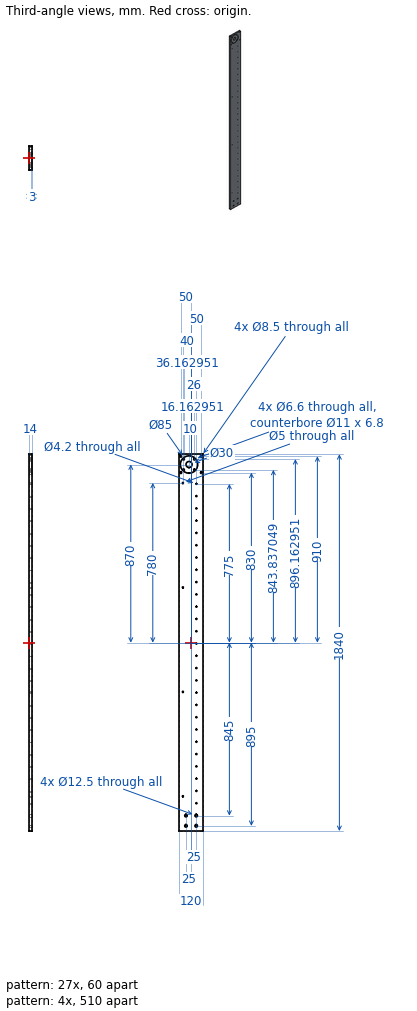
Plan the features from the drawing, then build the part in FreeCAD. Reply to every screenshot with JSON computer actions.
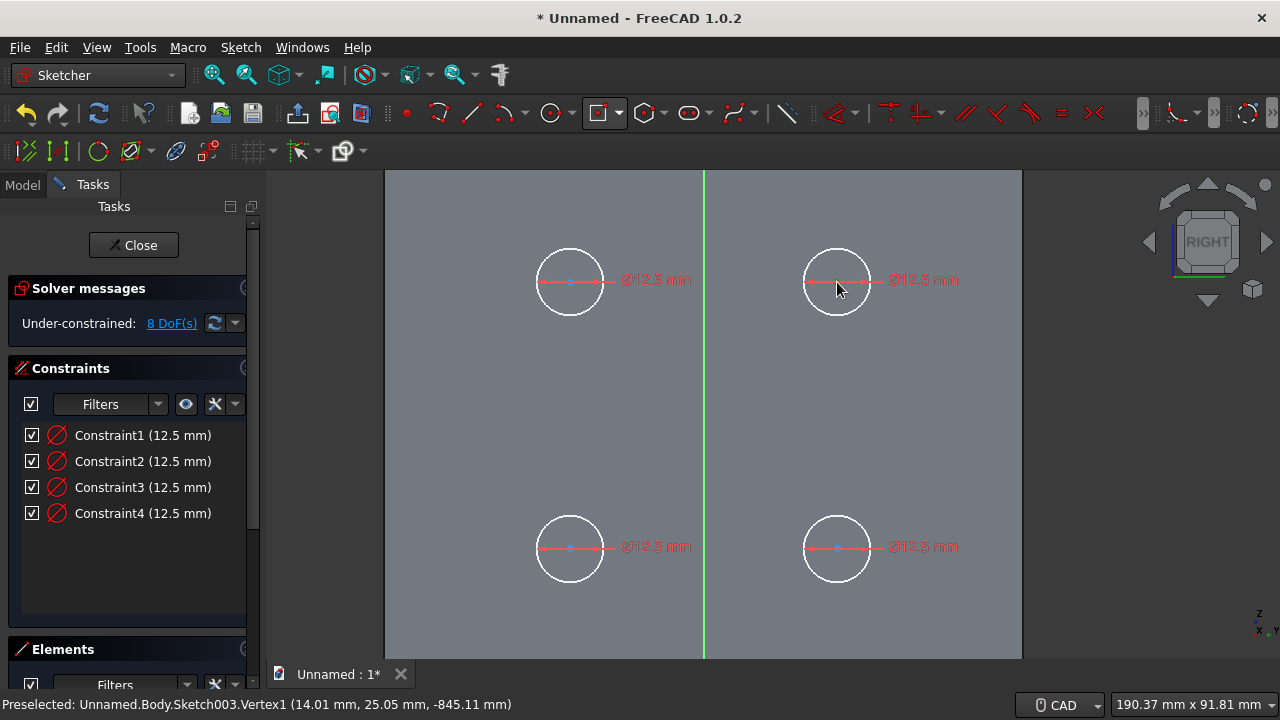
{"action": "left_click", "coordinate": [837, 549]}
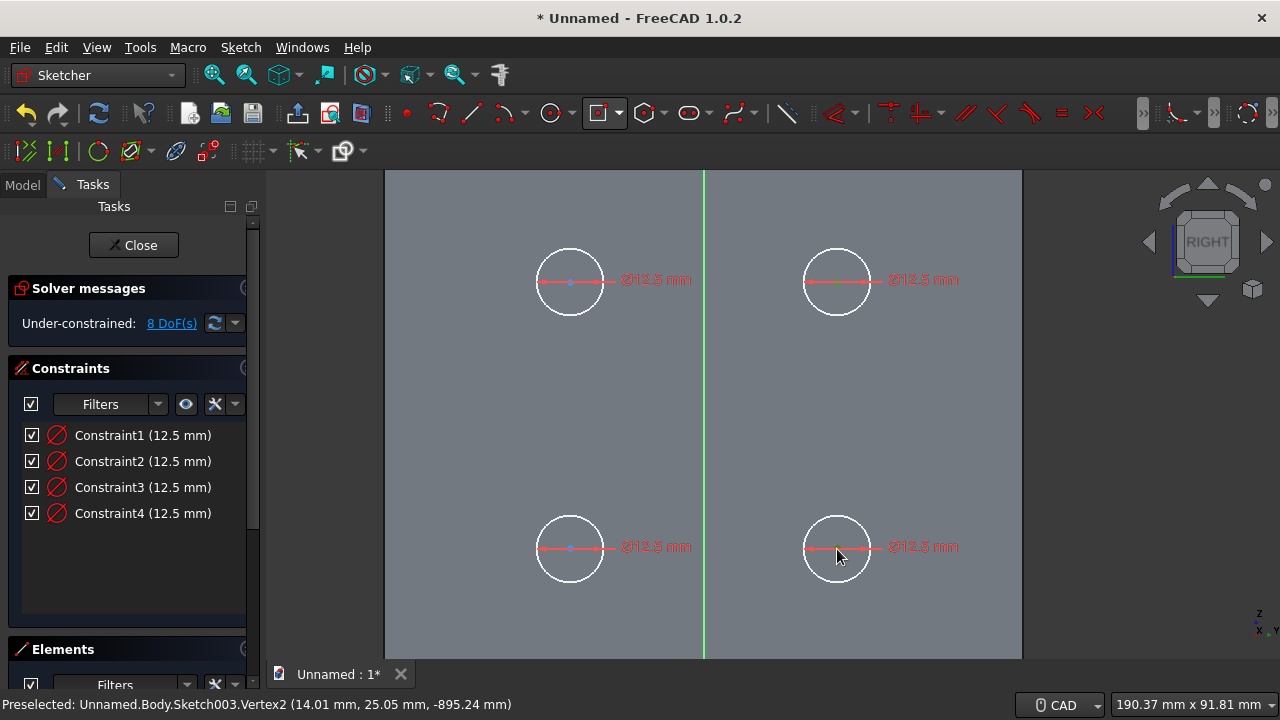
{"action": "left_click", "coordinate": [944, 114]}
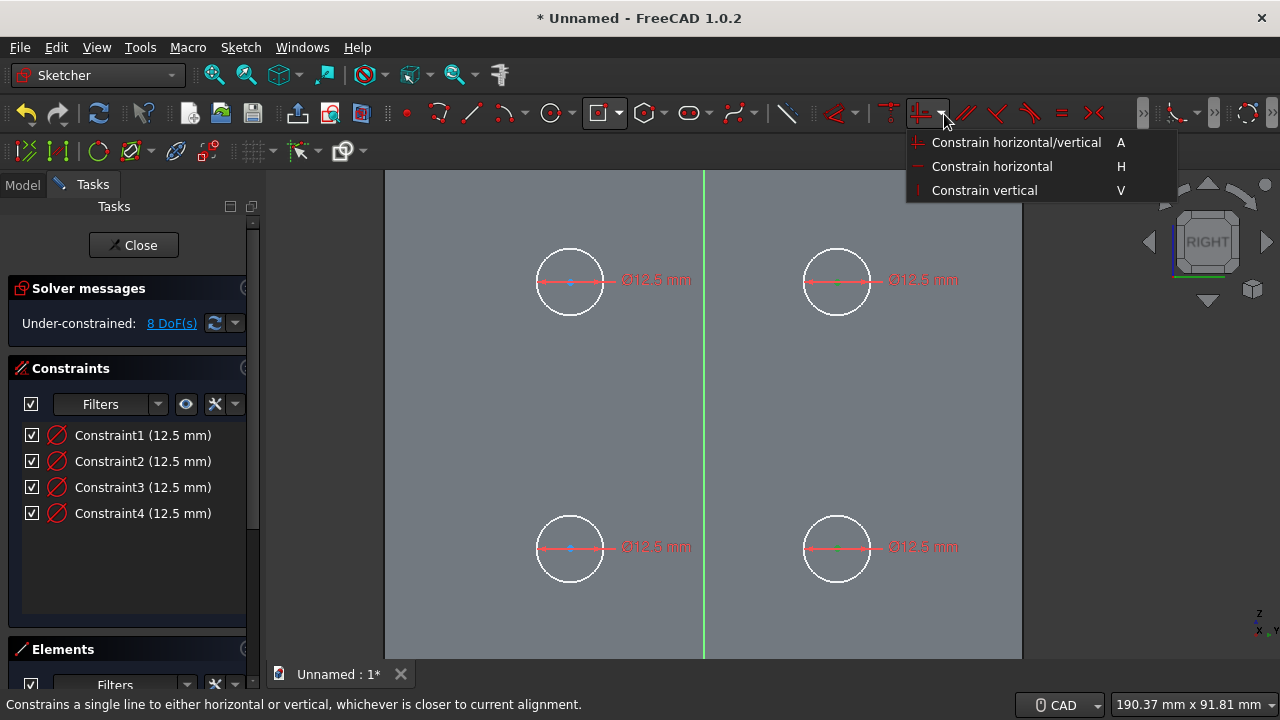
{"action": "left_click", "coordinate": [1042, 190]}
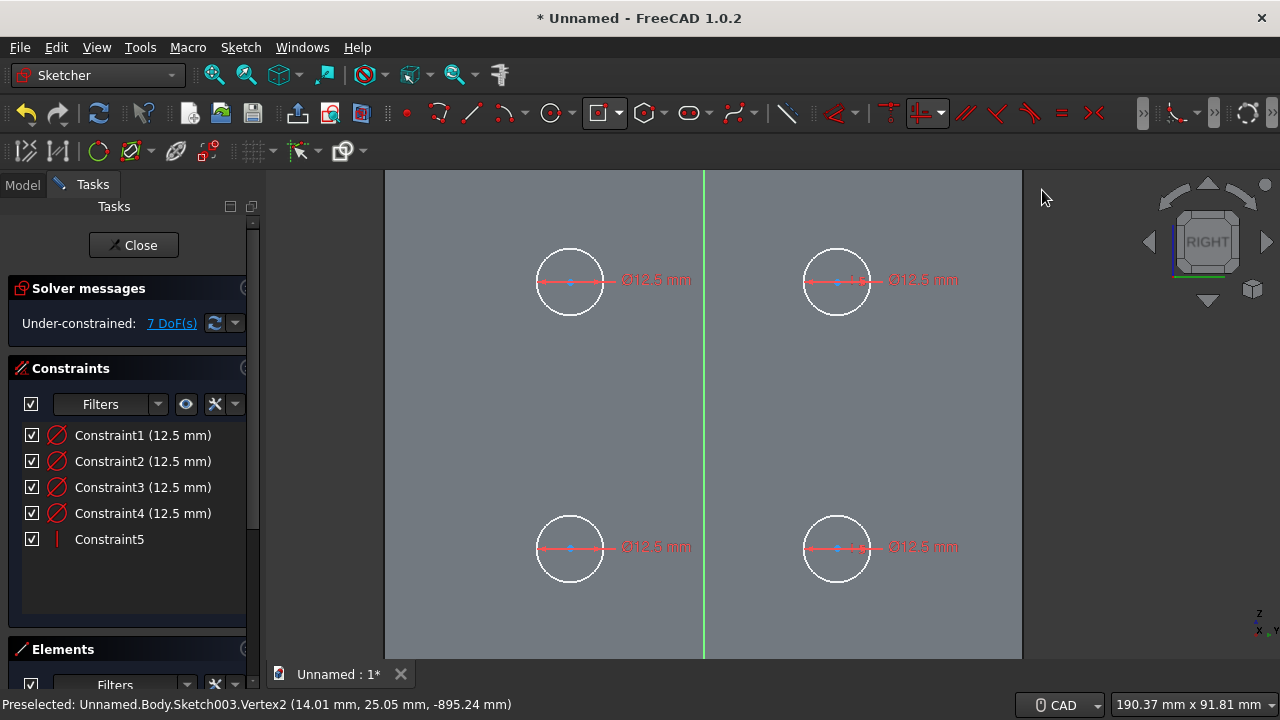
{"action": "left_click", "coordinate": [837, 282]}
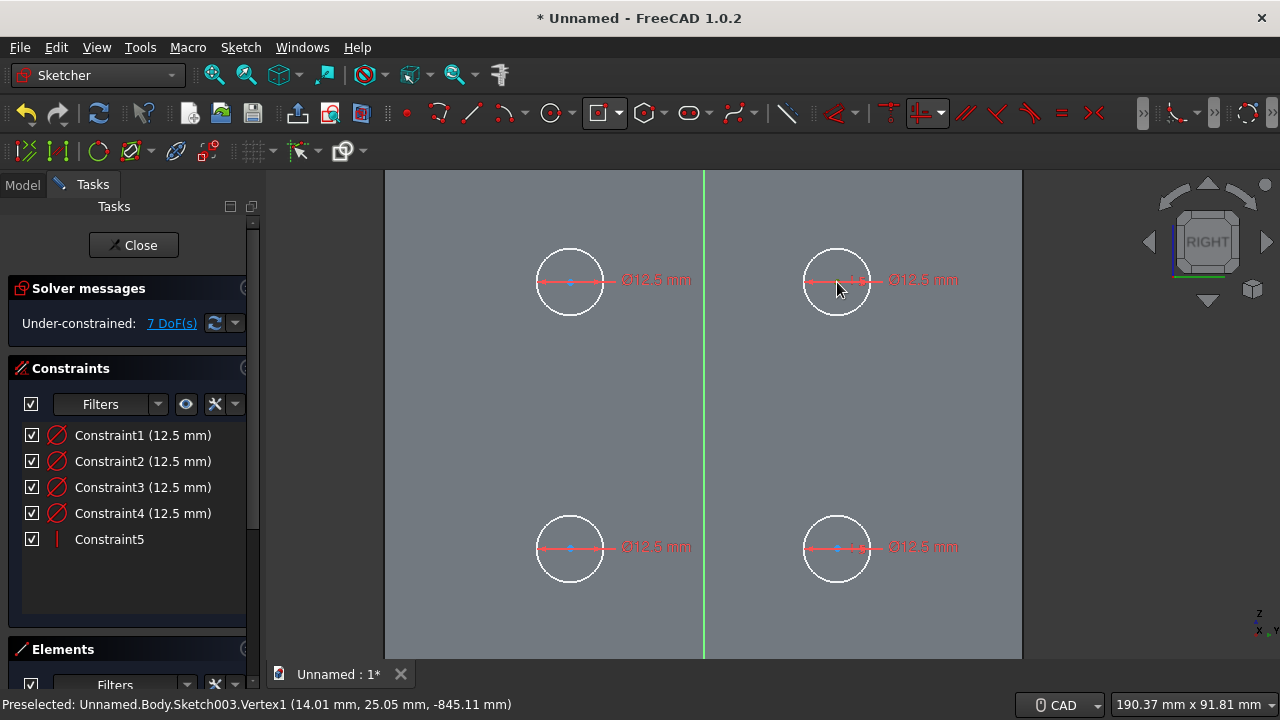
{"action": "left_click", "coordinate": [570, 282]}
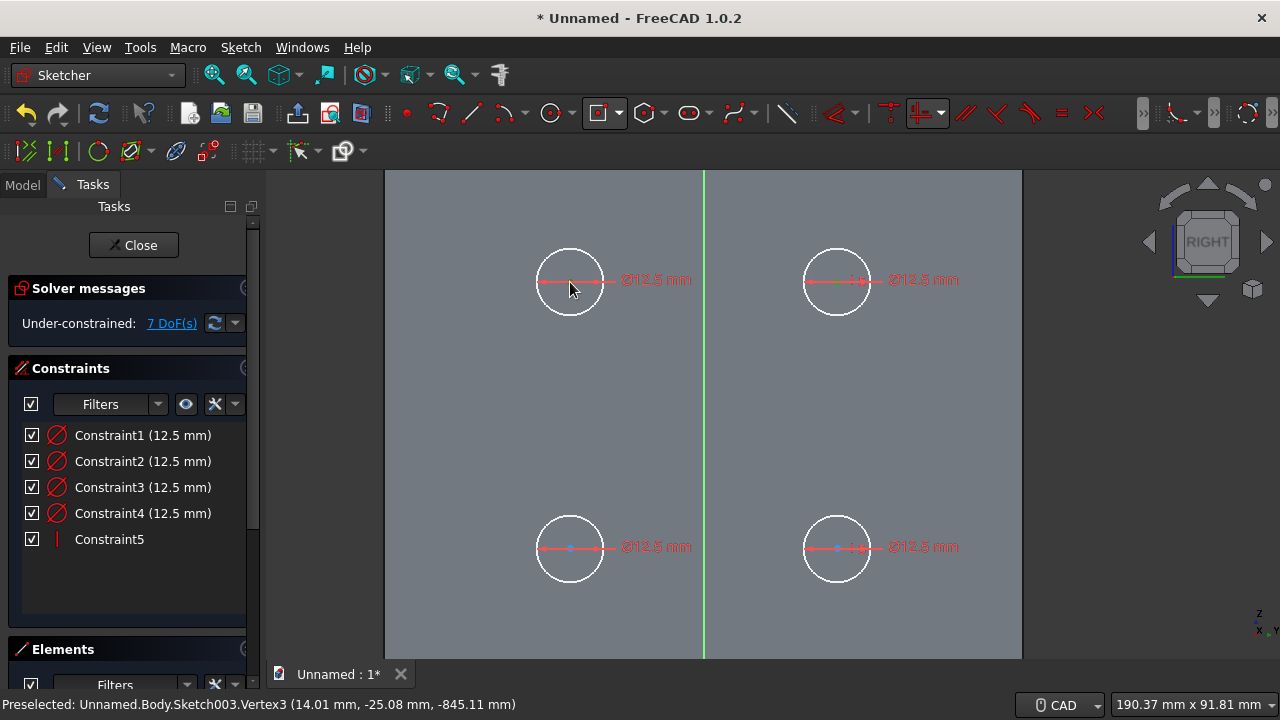
{"action": "key", "text": "h"}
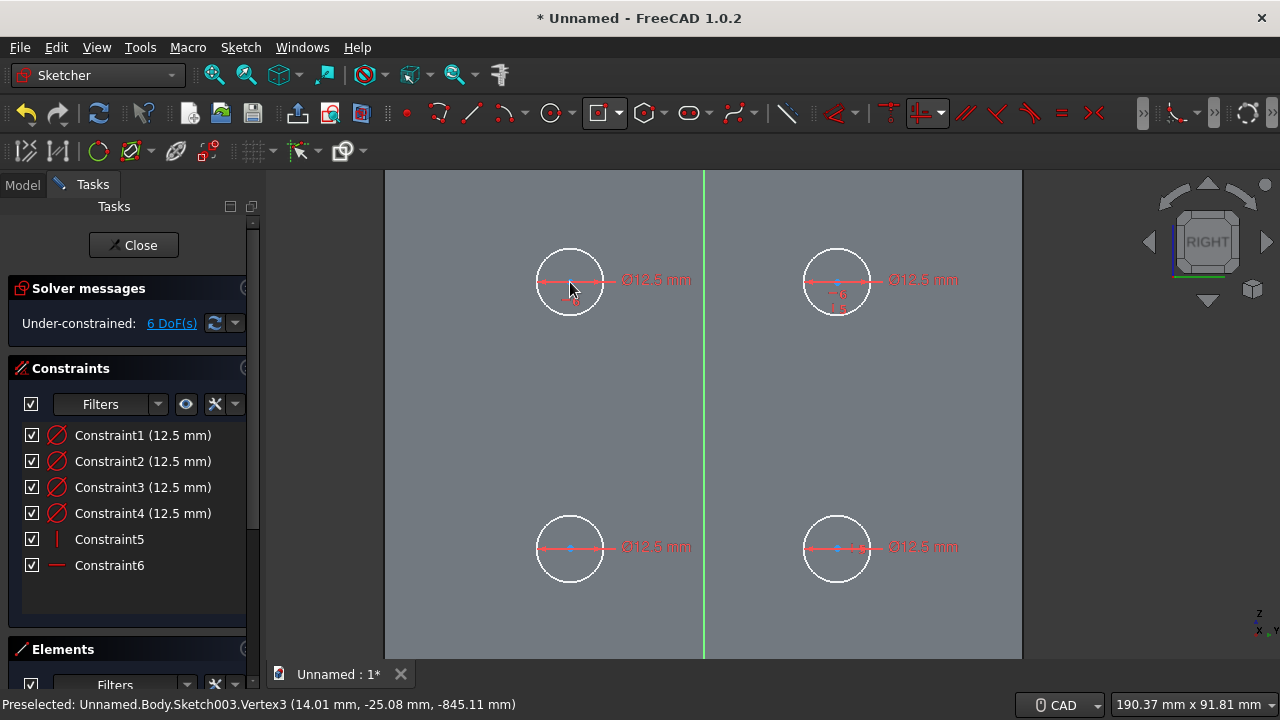
{"action": "left_click", "coordinate": [570, 282]}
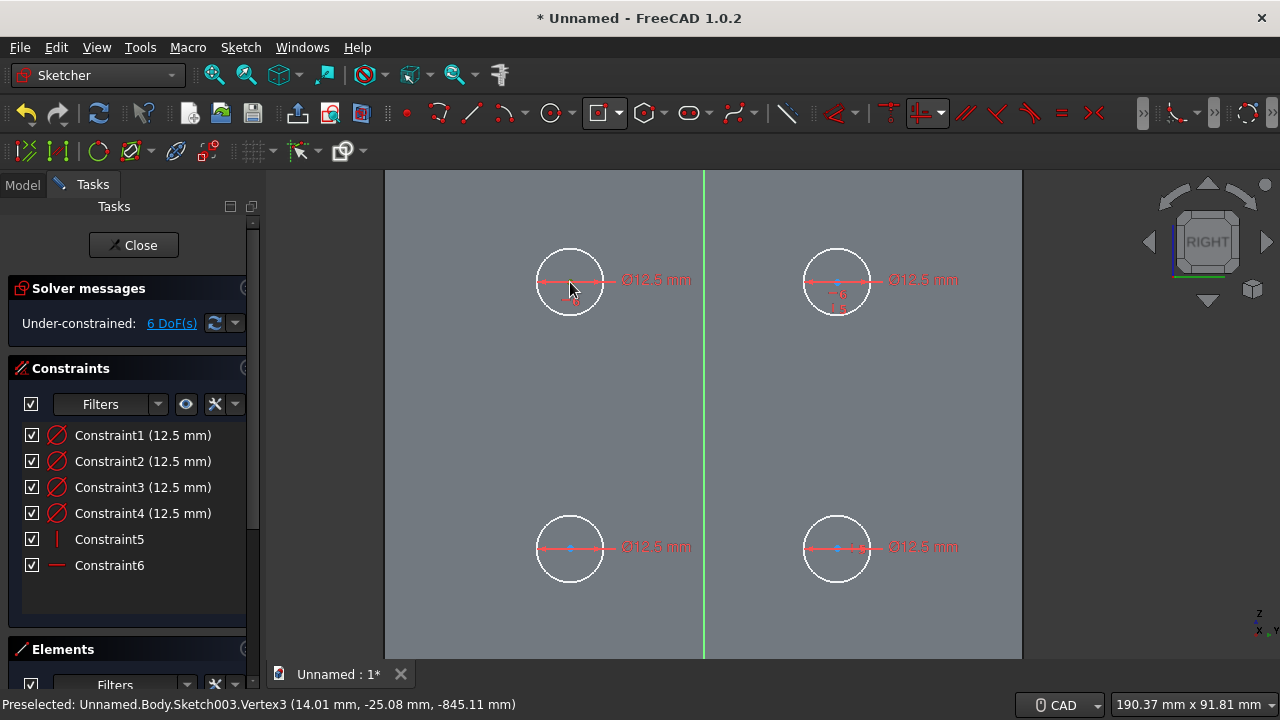
{"action": "left_click", "coordinate": [570, 549]}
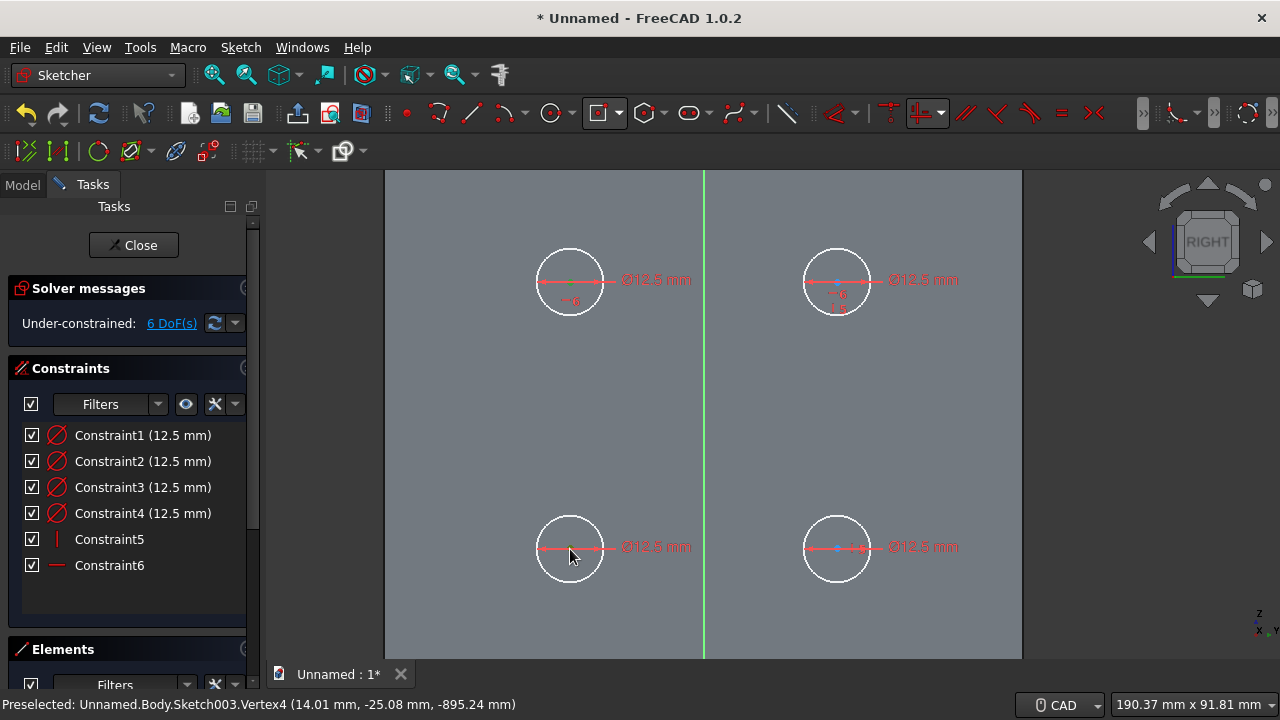
{"action": "key", "text": "v"}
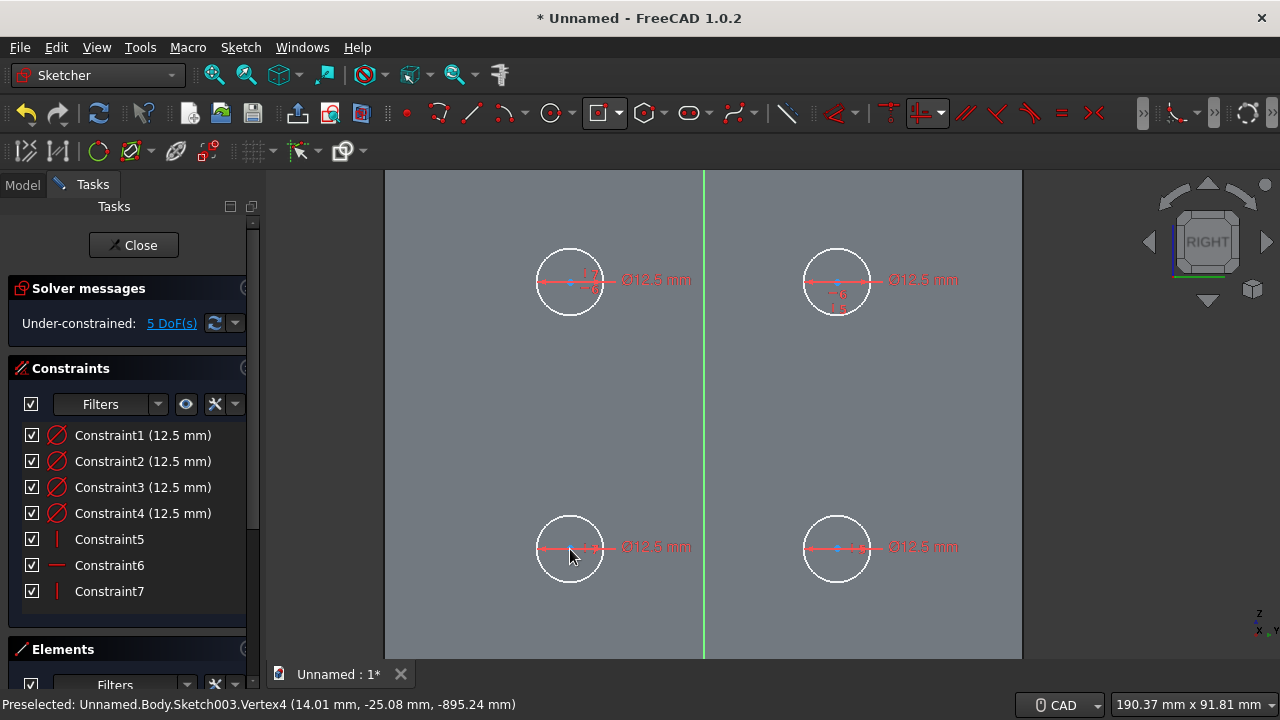
{"action": "left_click", "coordinate": [837, 549]}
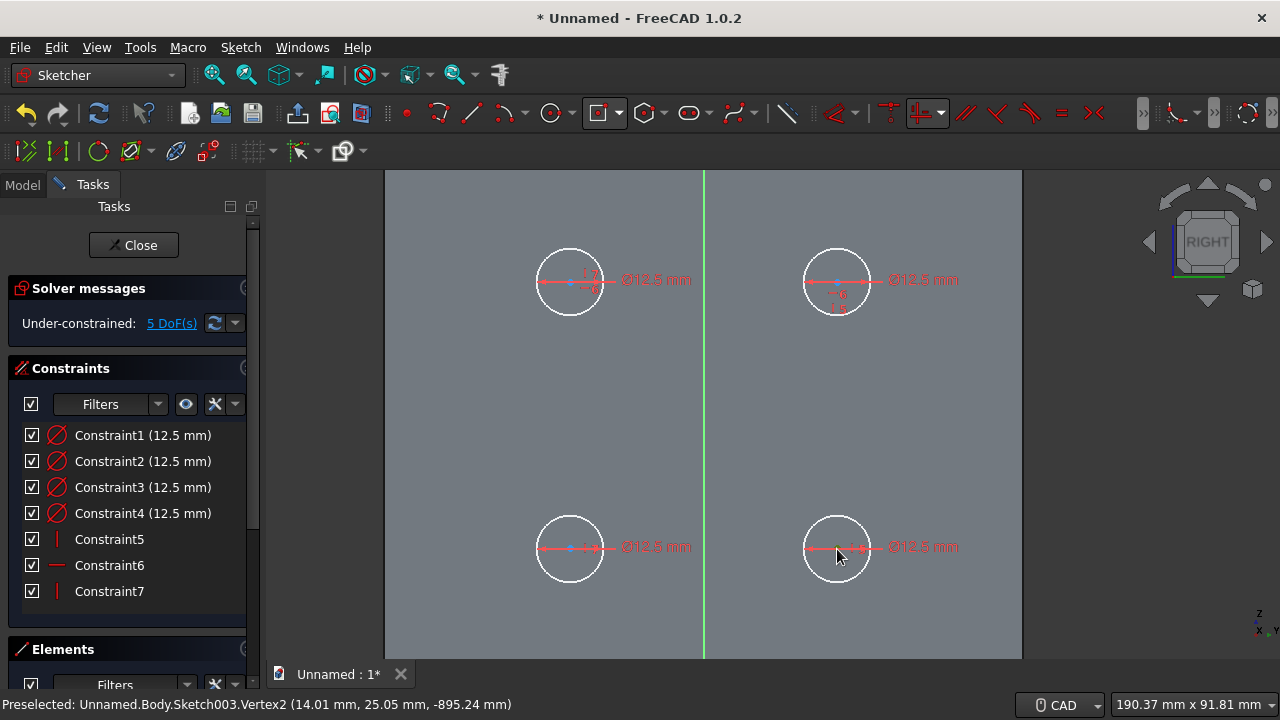
{"action": "left_click", "coordinate": [570, 549]}